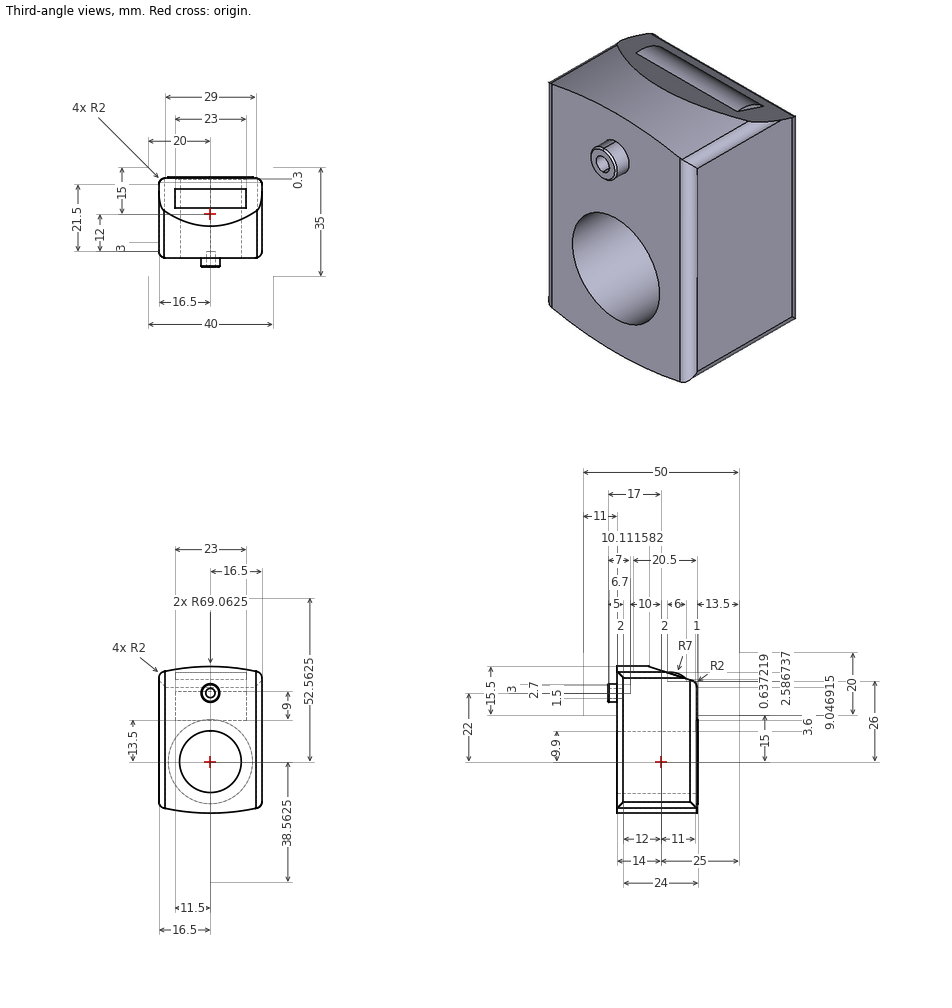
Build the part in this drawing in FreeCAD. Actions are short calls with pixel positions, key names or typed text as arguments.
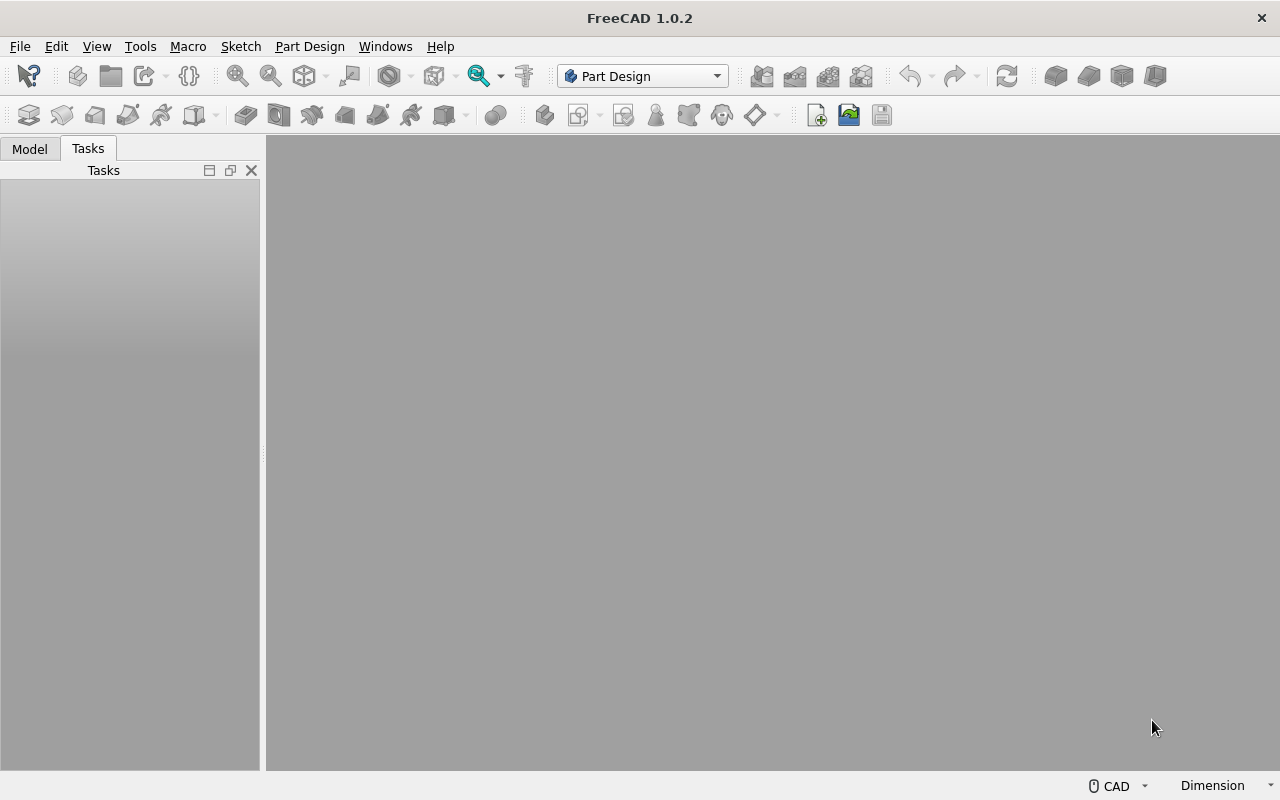
click(816, 116)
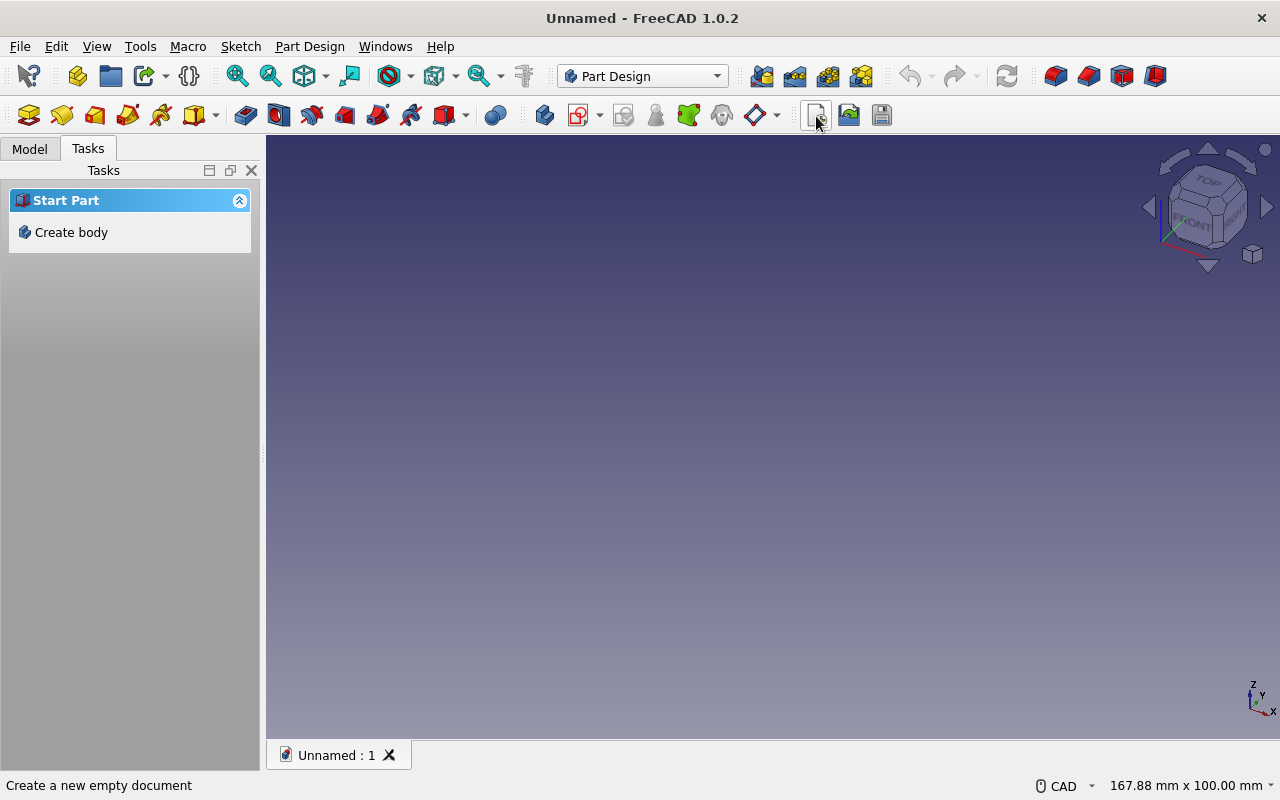
click(545, 116)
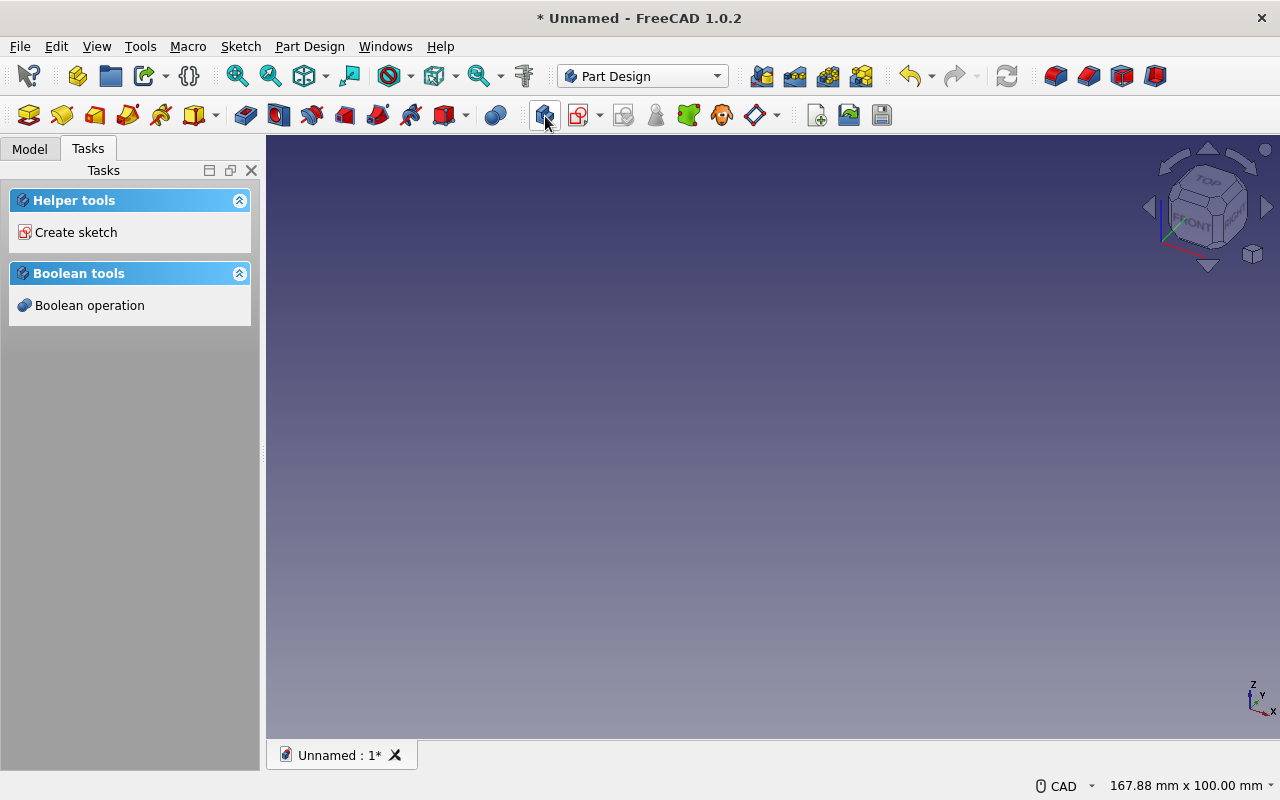
click(30, 148)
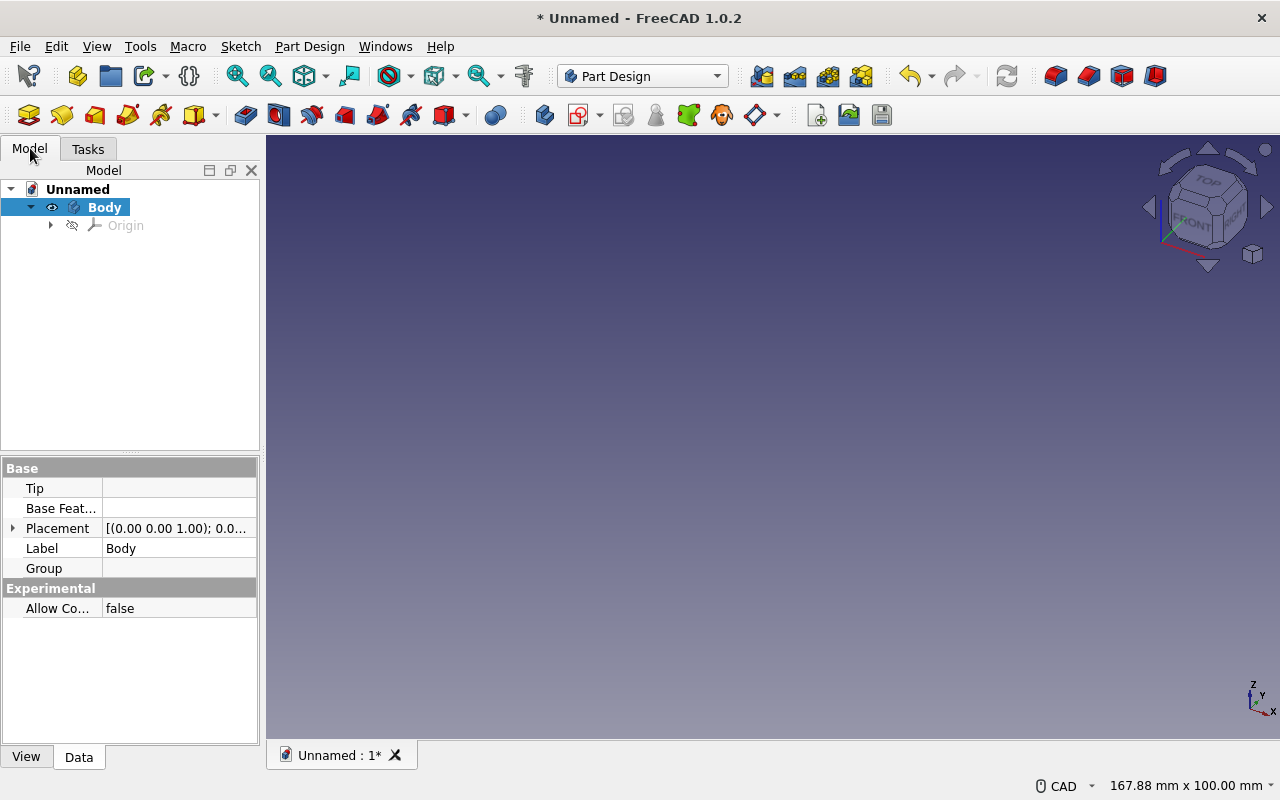
click(51, 225)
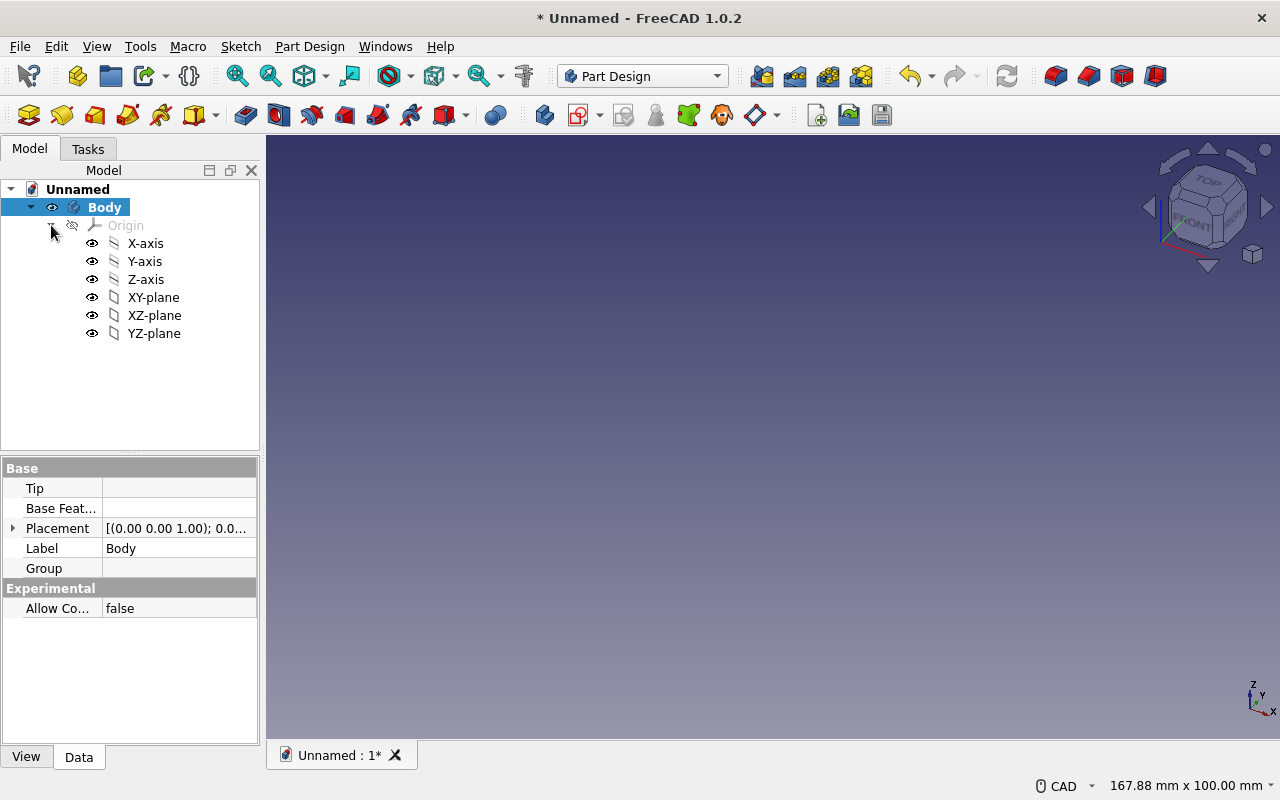
click(137, 315)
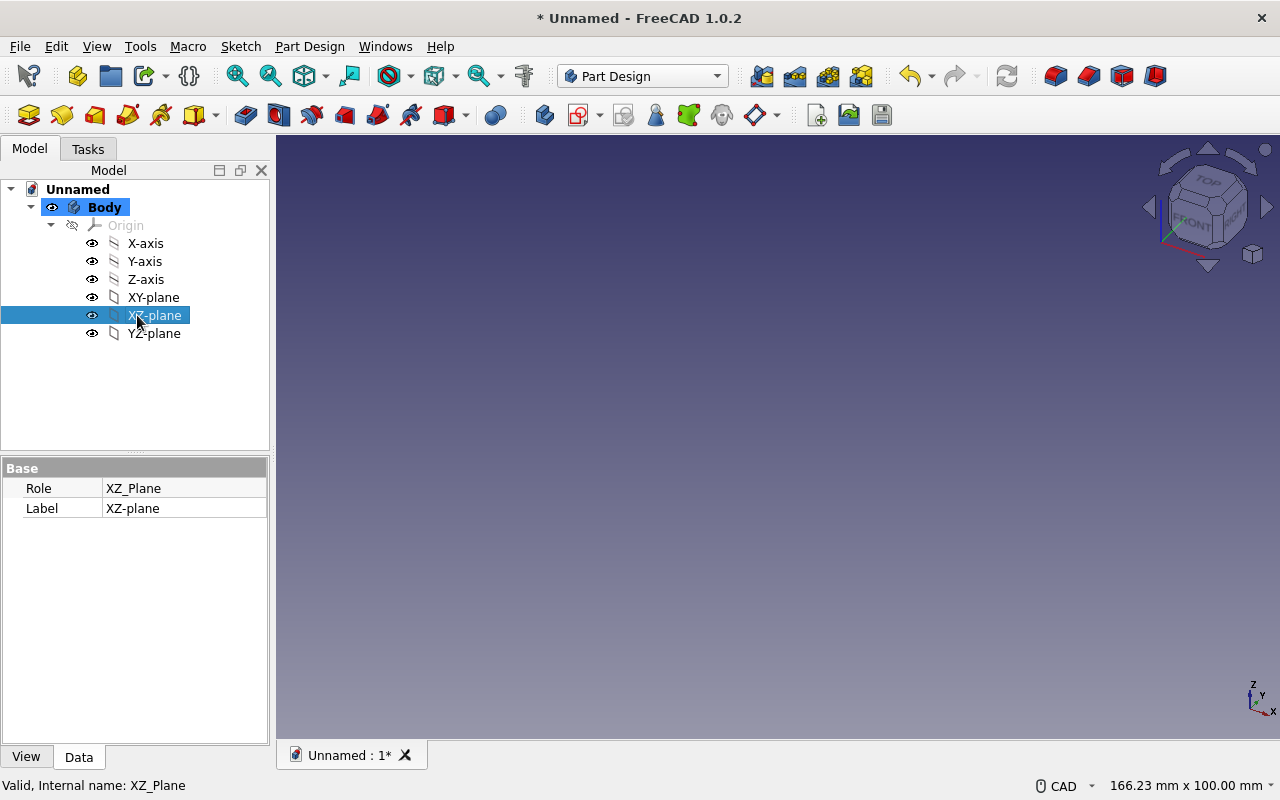
click(754, 116)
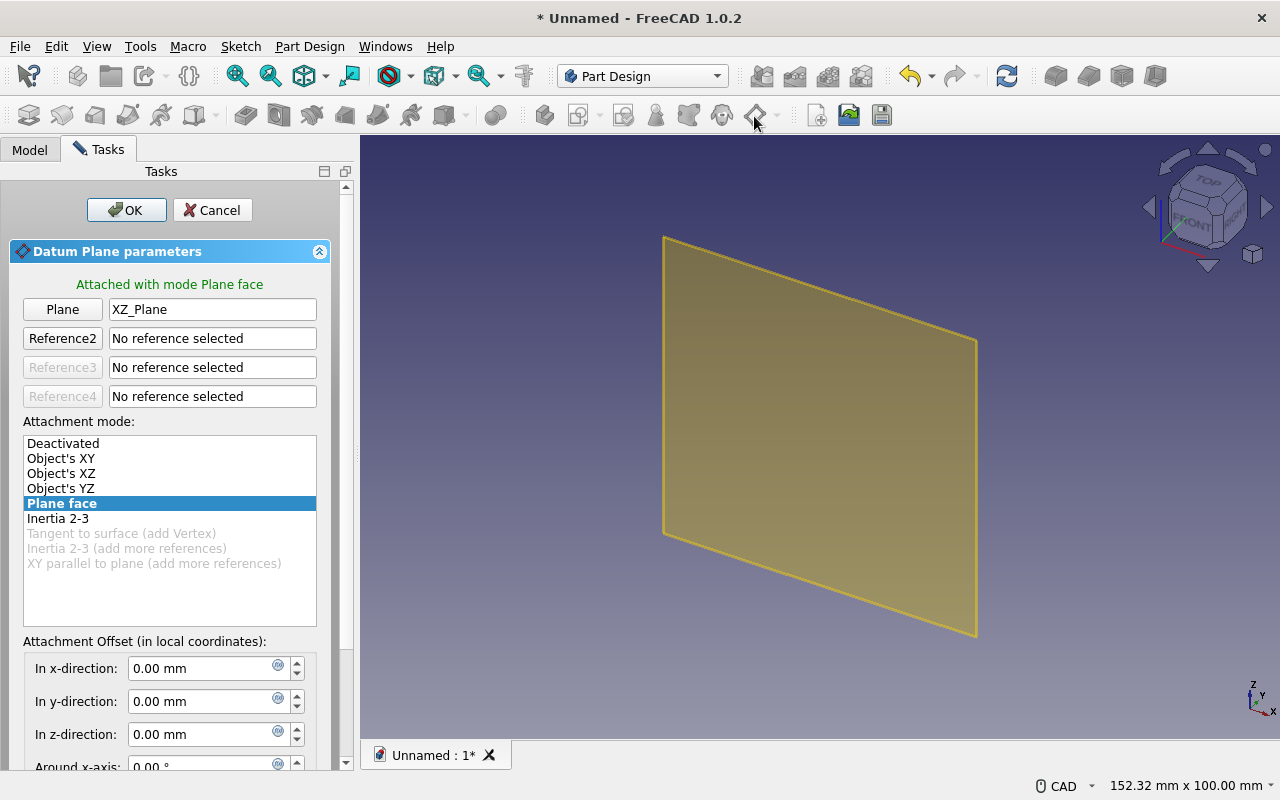
triple_click(210, 734)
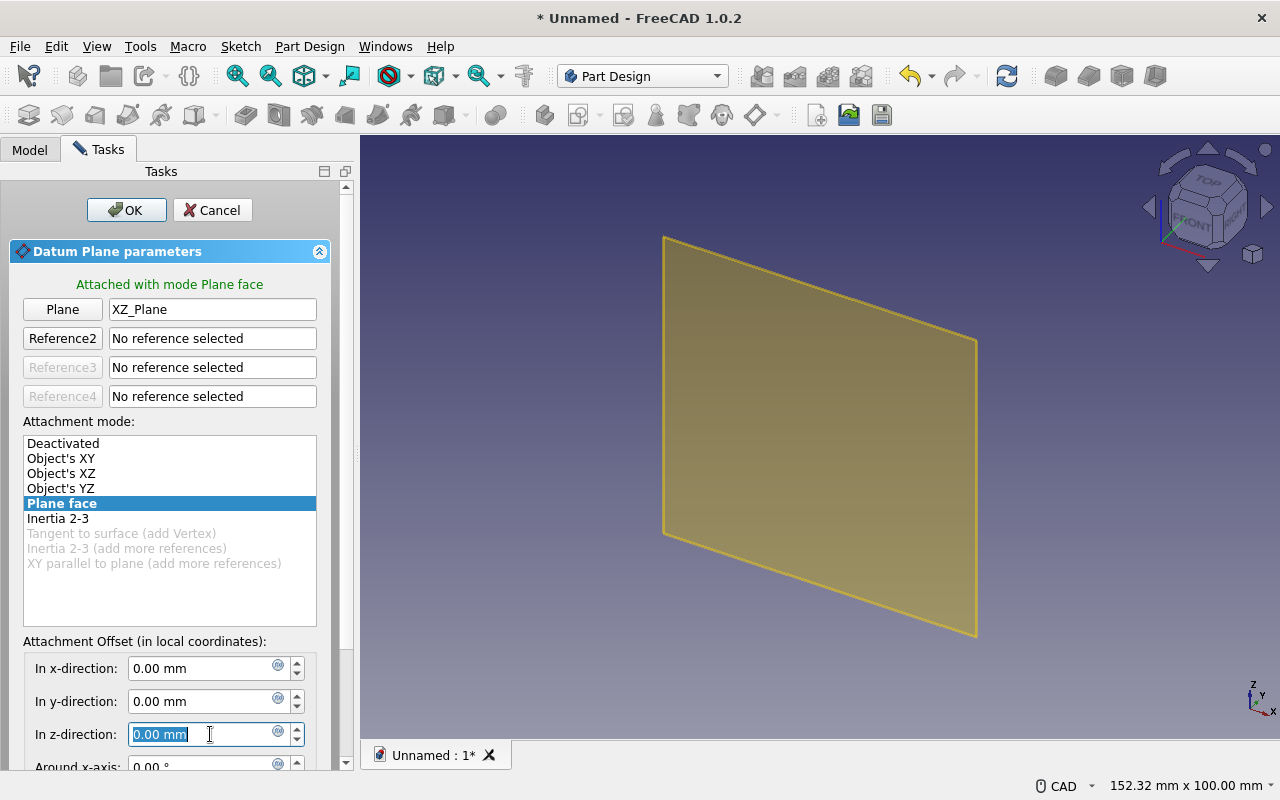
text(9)
key(Tab)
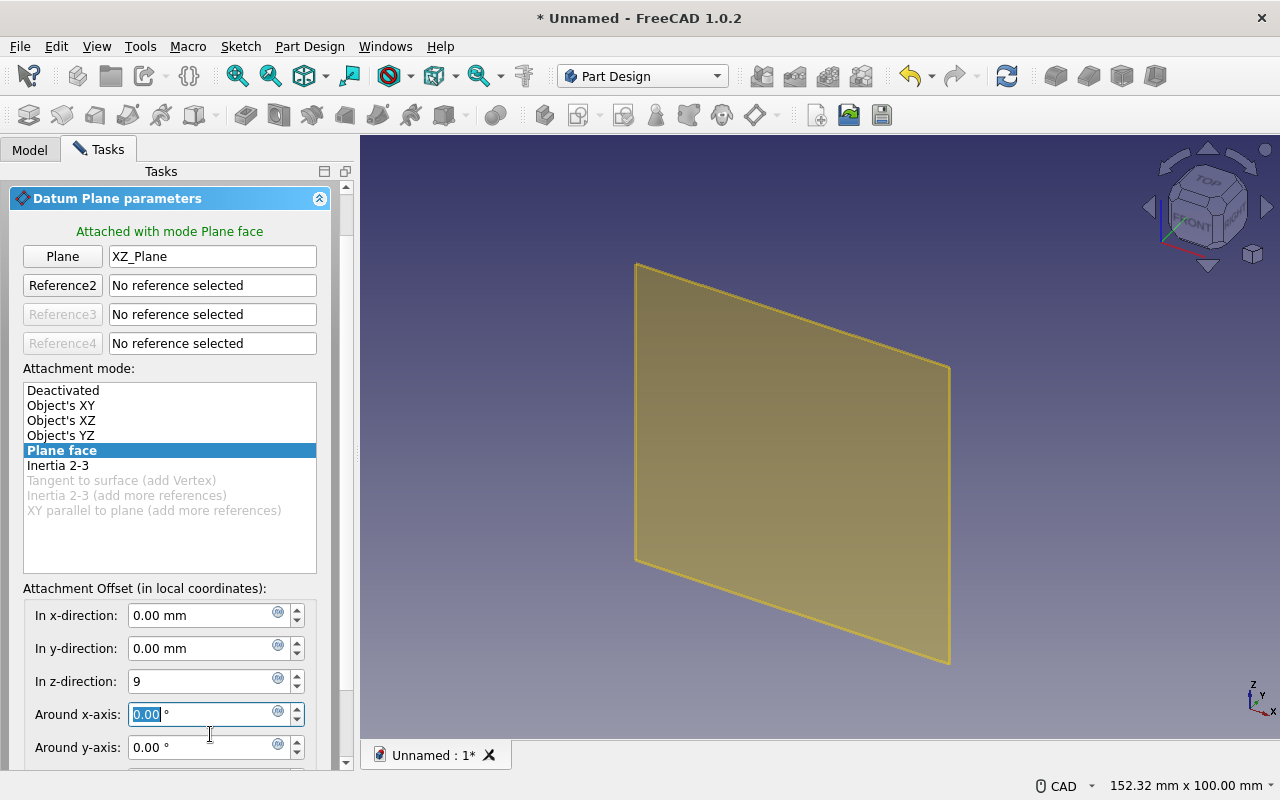
scroll(346, 476, up, 2)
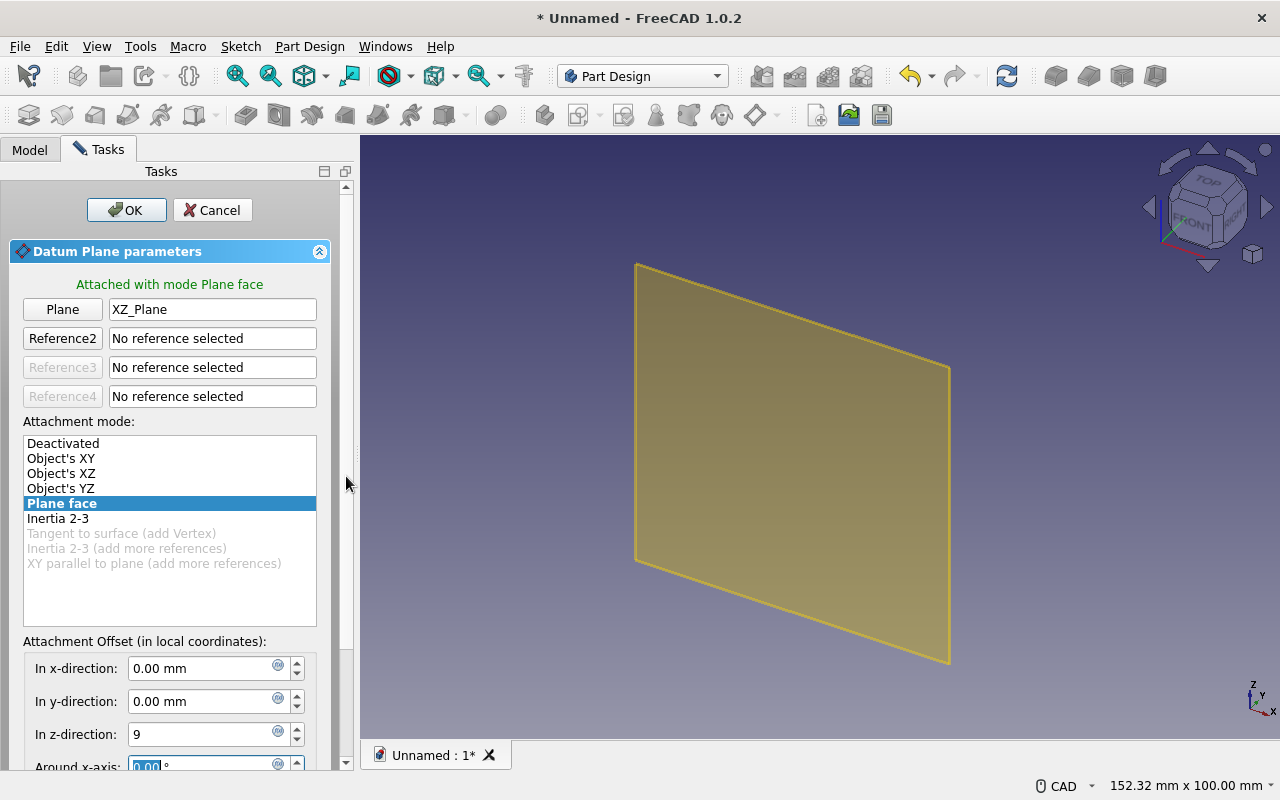
click(127, 210)